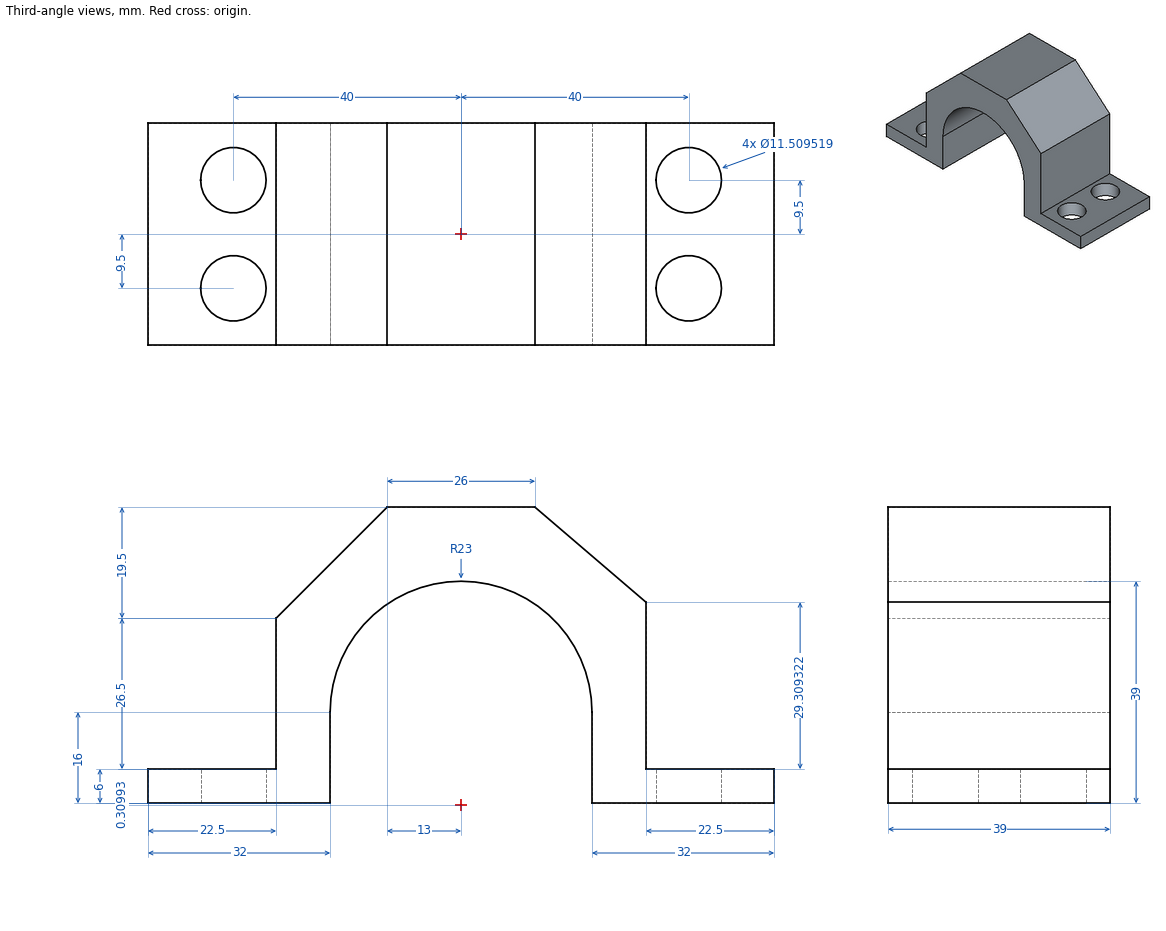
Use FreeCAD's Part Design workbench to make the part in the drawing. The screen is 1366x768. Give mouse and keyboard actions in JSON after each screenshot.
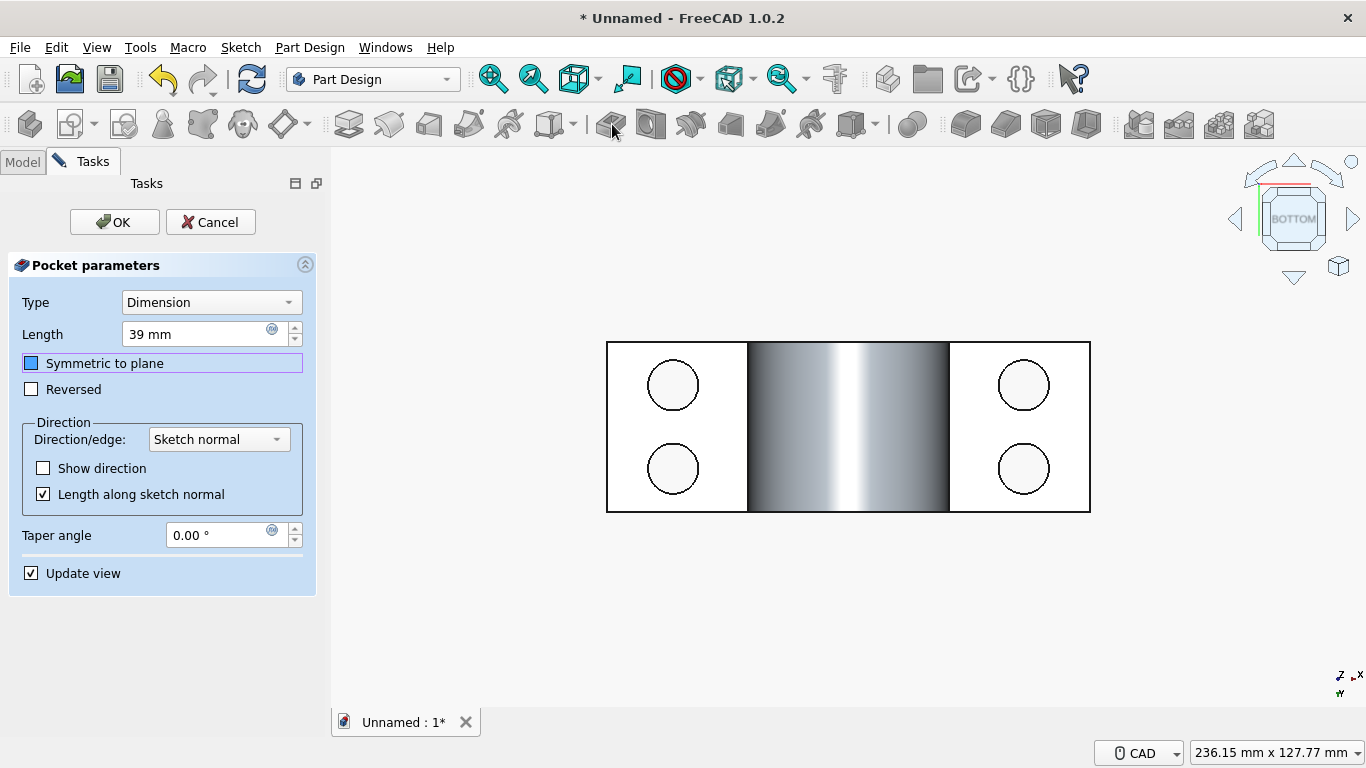
{"action": "left_click", "coordinate": [115, 222]}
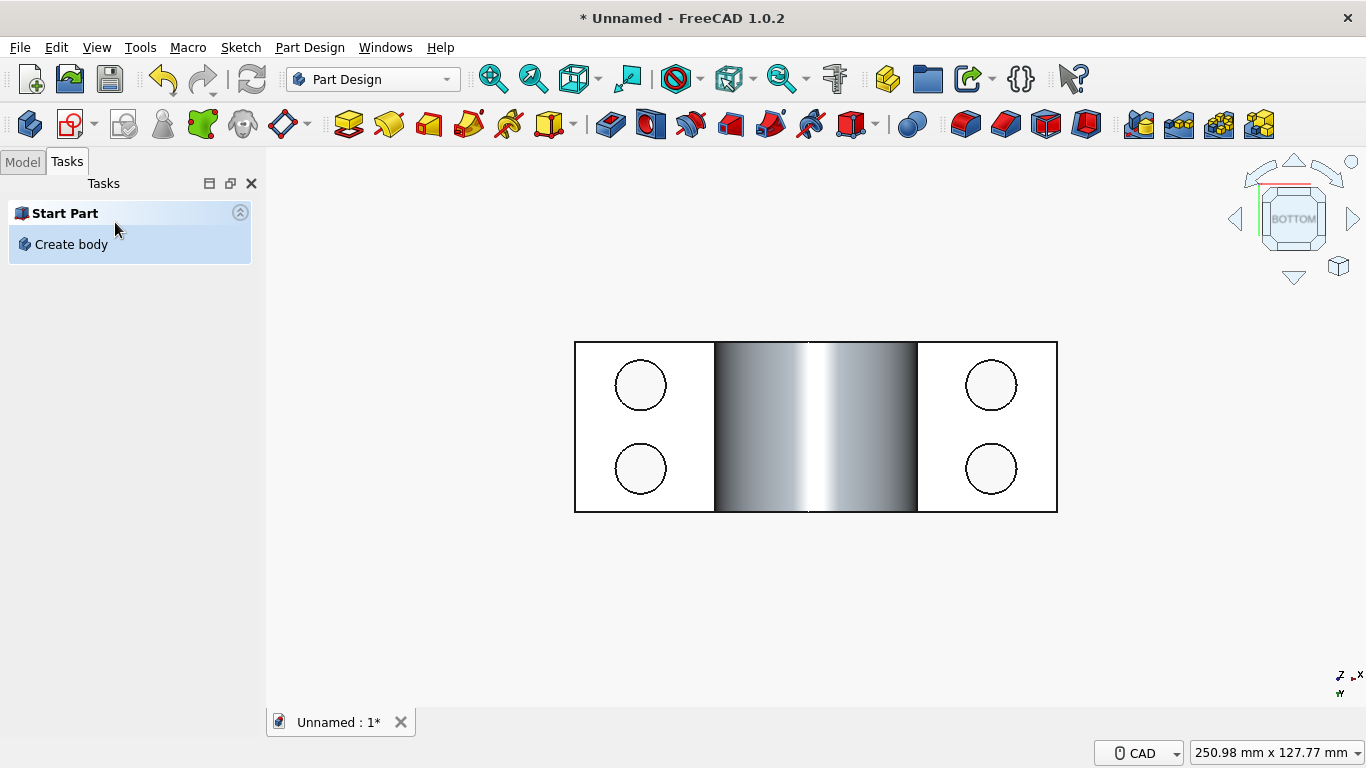
{"action": "key", "text": "0"}